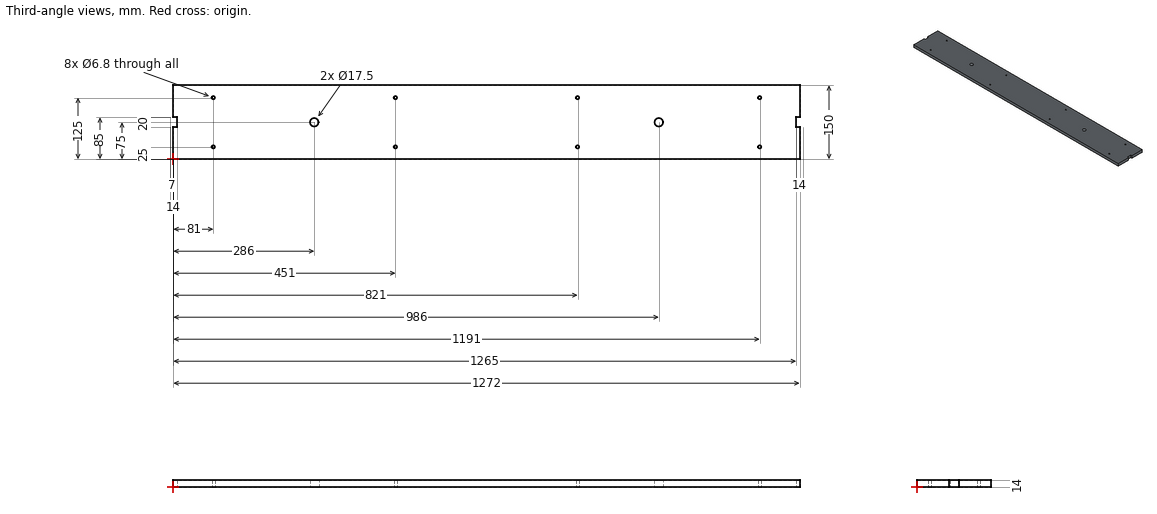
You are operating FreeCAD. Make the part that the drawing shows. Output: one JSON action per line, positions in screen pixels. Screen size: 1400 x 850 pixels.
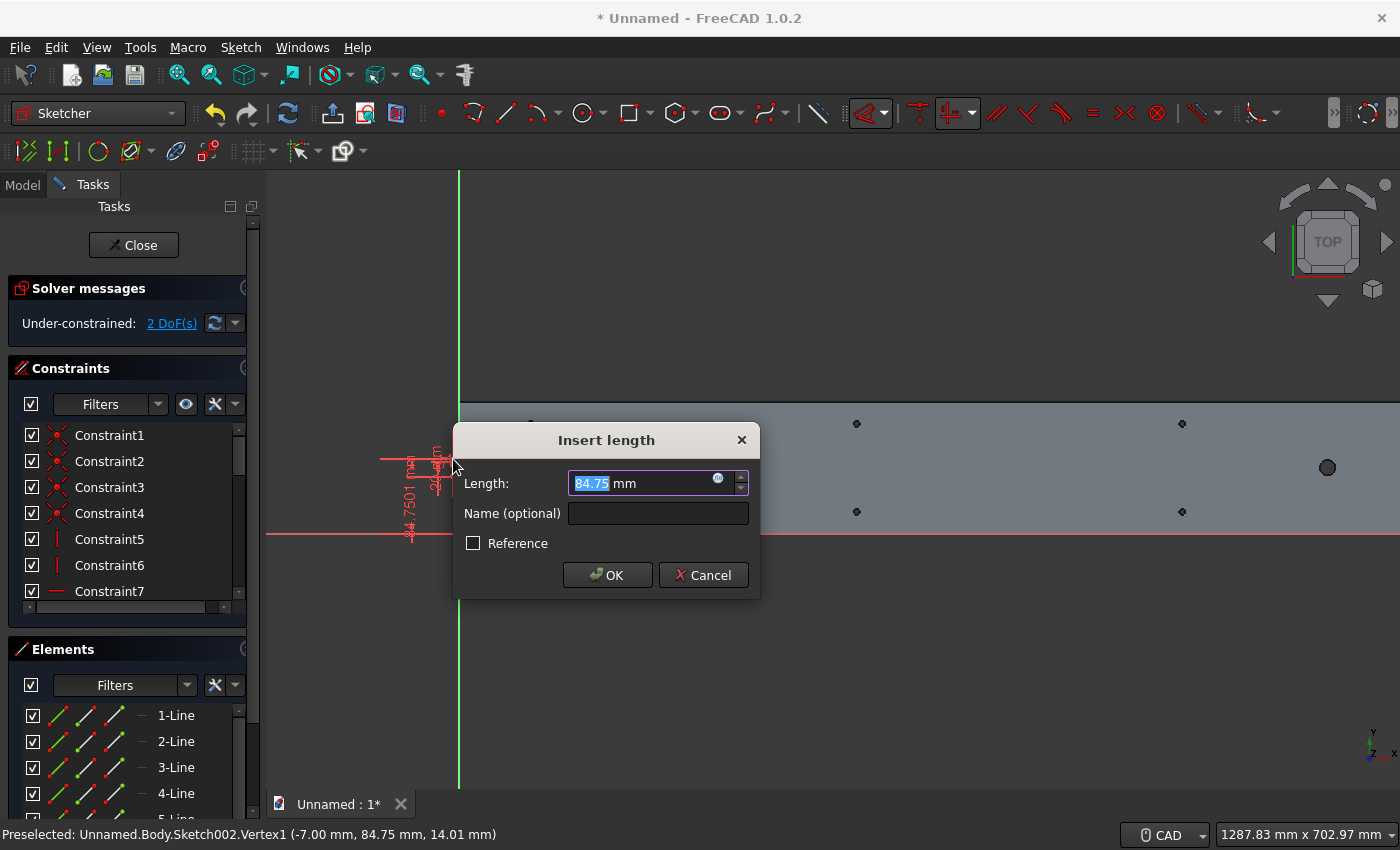
{"action": "type", "text": "85"}
{"action": "key", "text": "Return"}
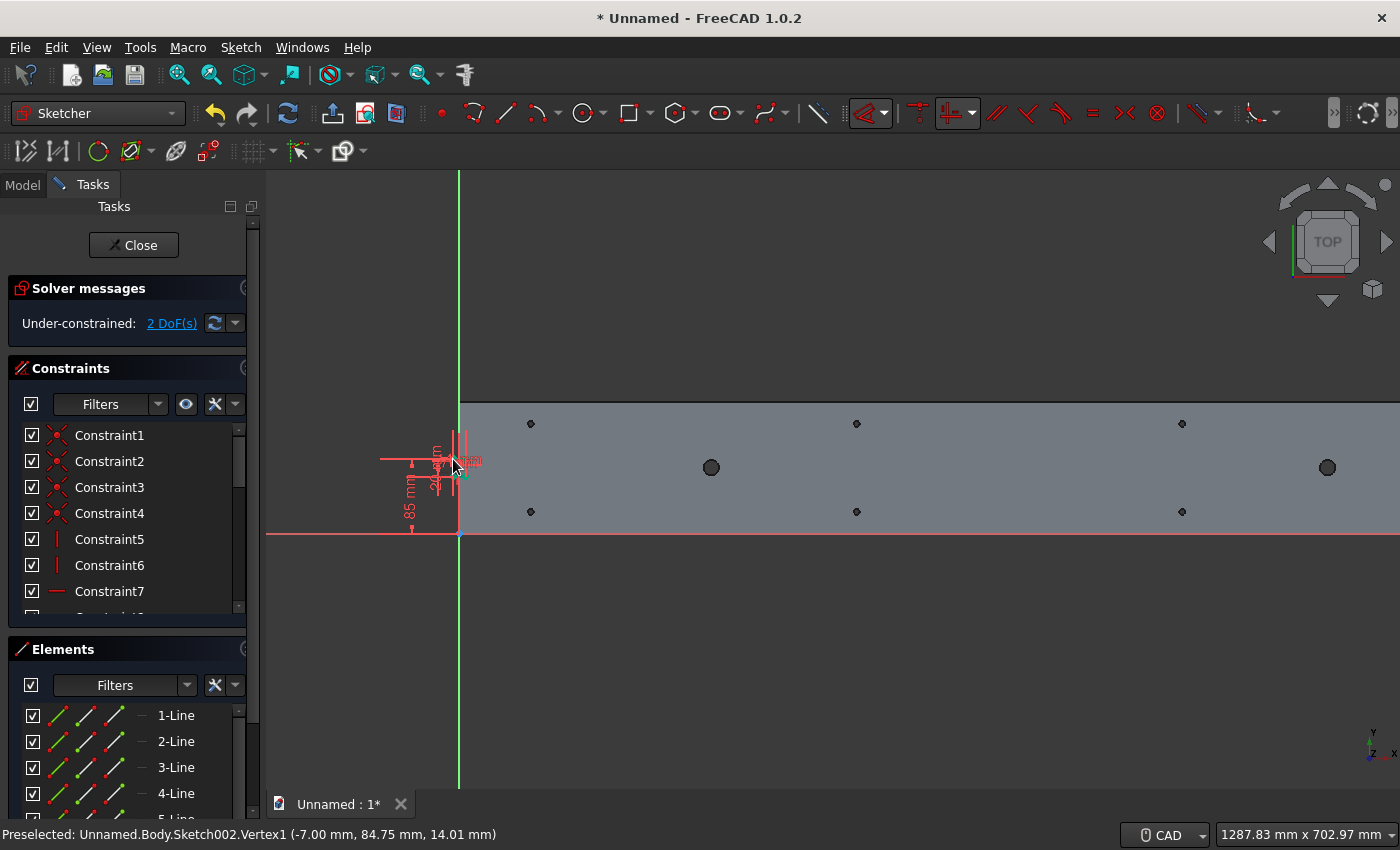
{"action": "scroll", "coordinate": [454, 459], "scroll_direction": "down", "scroll_amount": 3}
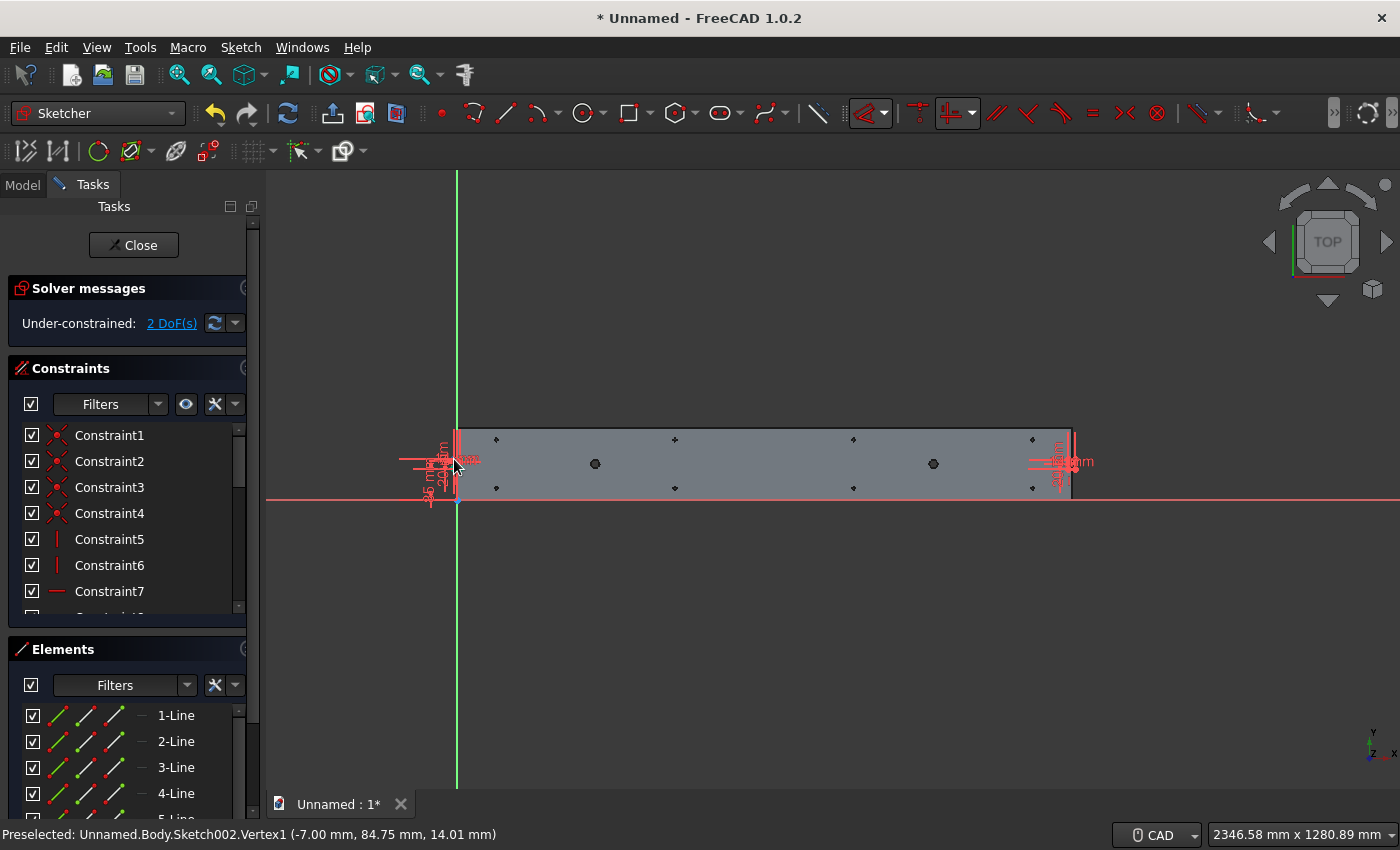
{"action": "scroll", "coordinate": [1068, 460], "scroll_direction": "up", "scroll_amount": 3}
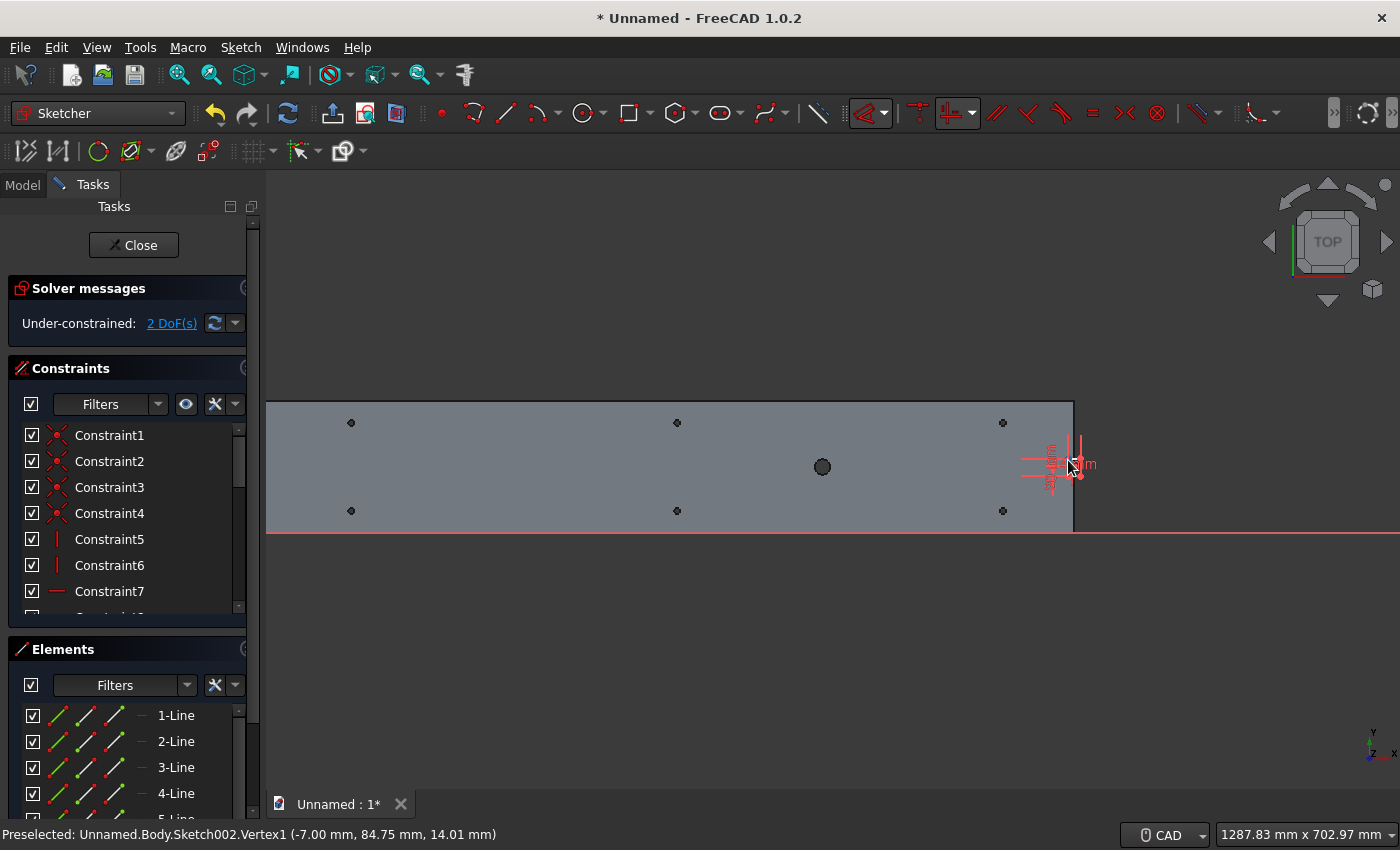
{"action": "left_click", "coordinate": [1068, 459]}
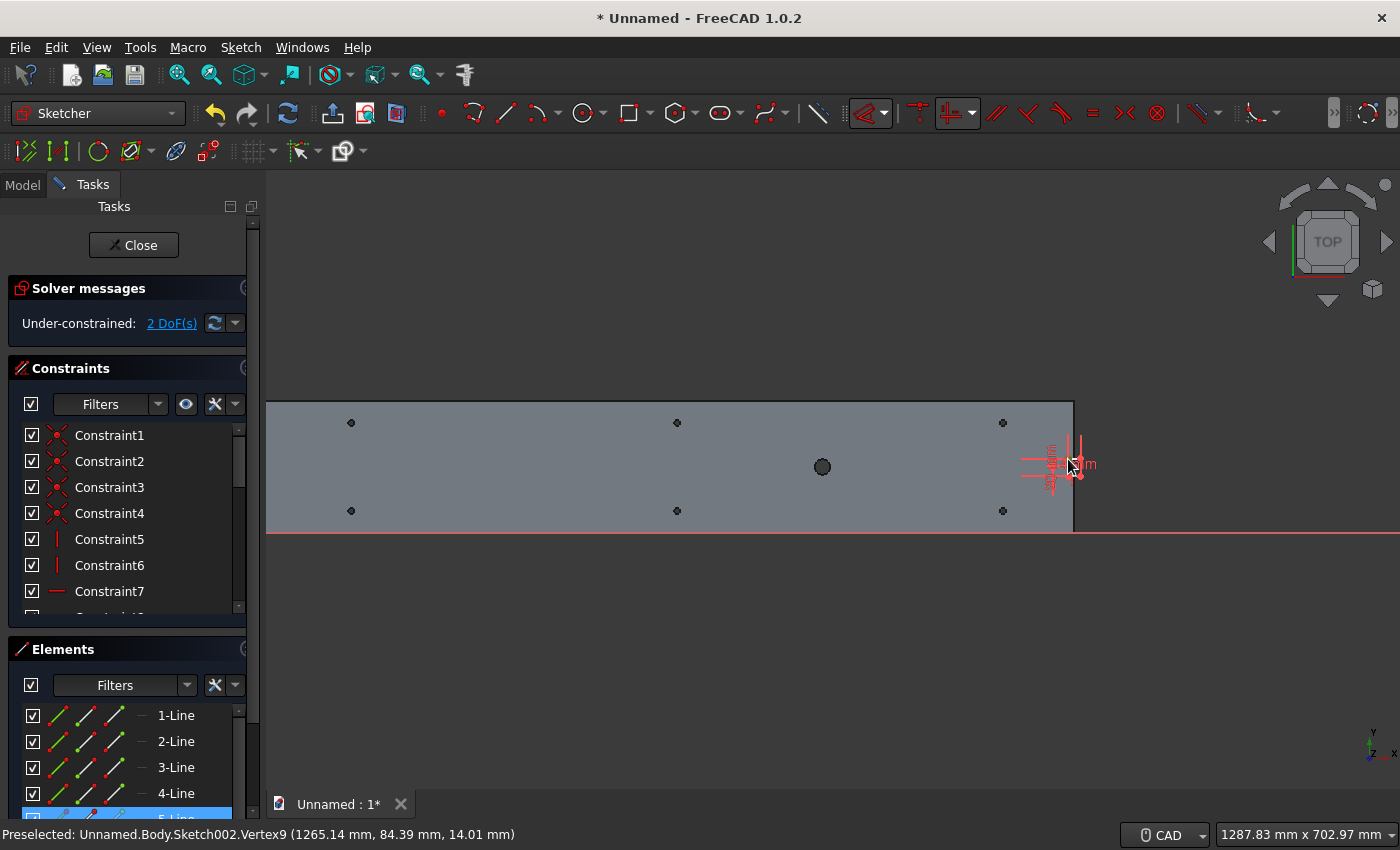
{"action": "left_click", "coordinate": [886, 114]}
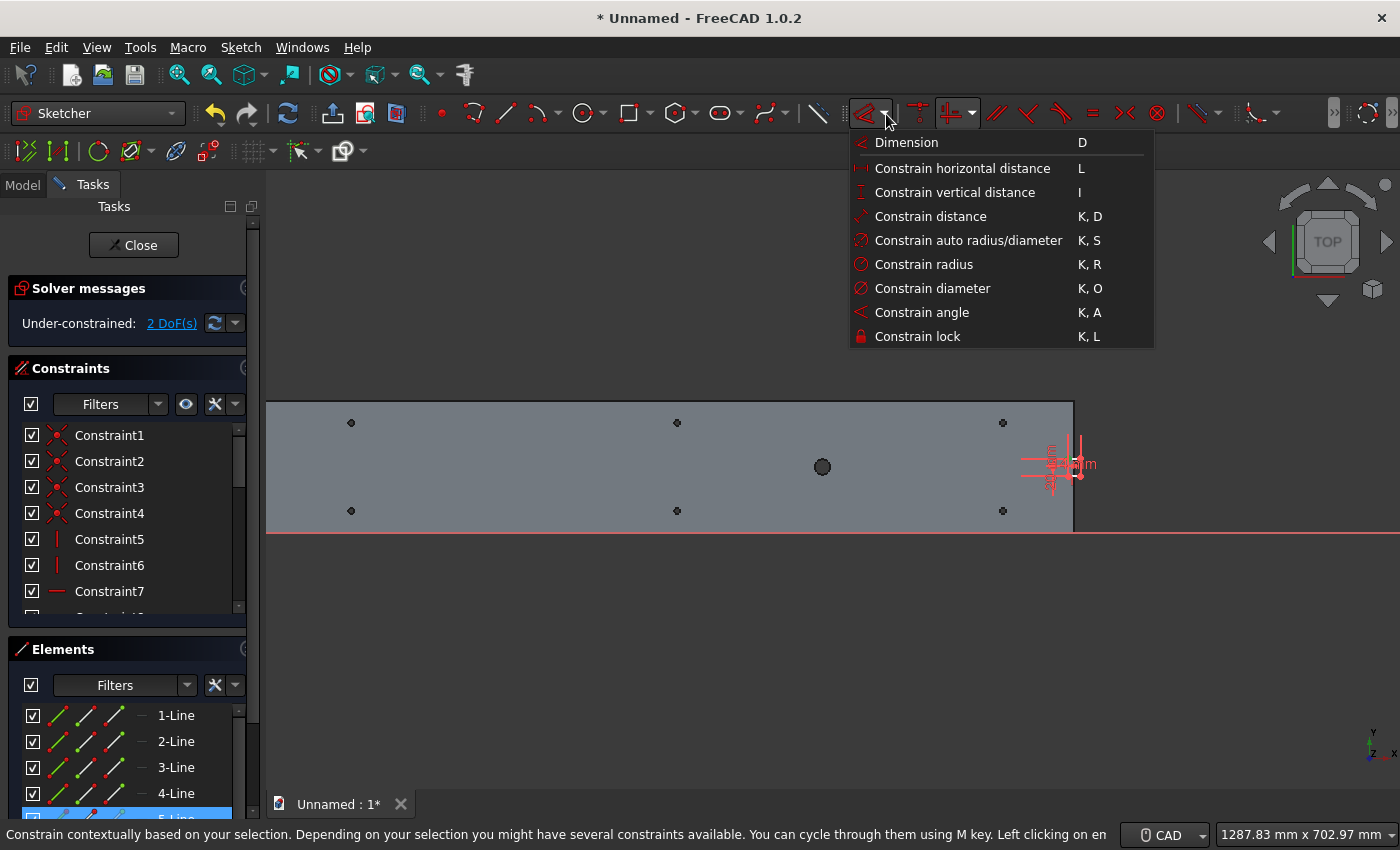
{"action": "left_click", "coordinate": [1002, 192]}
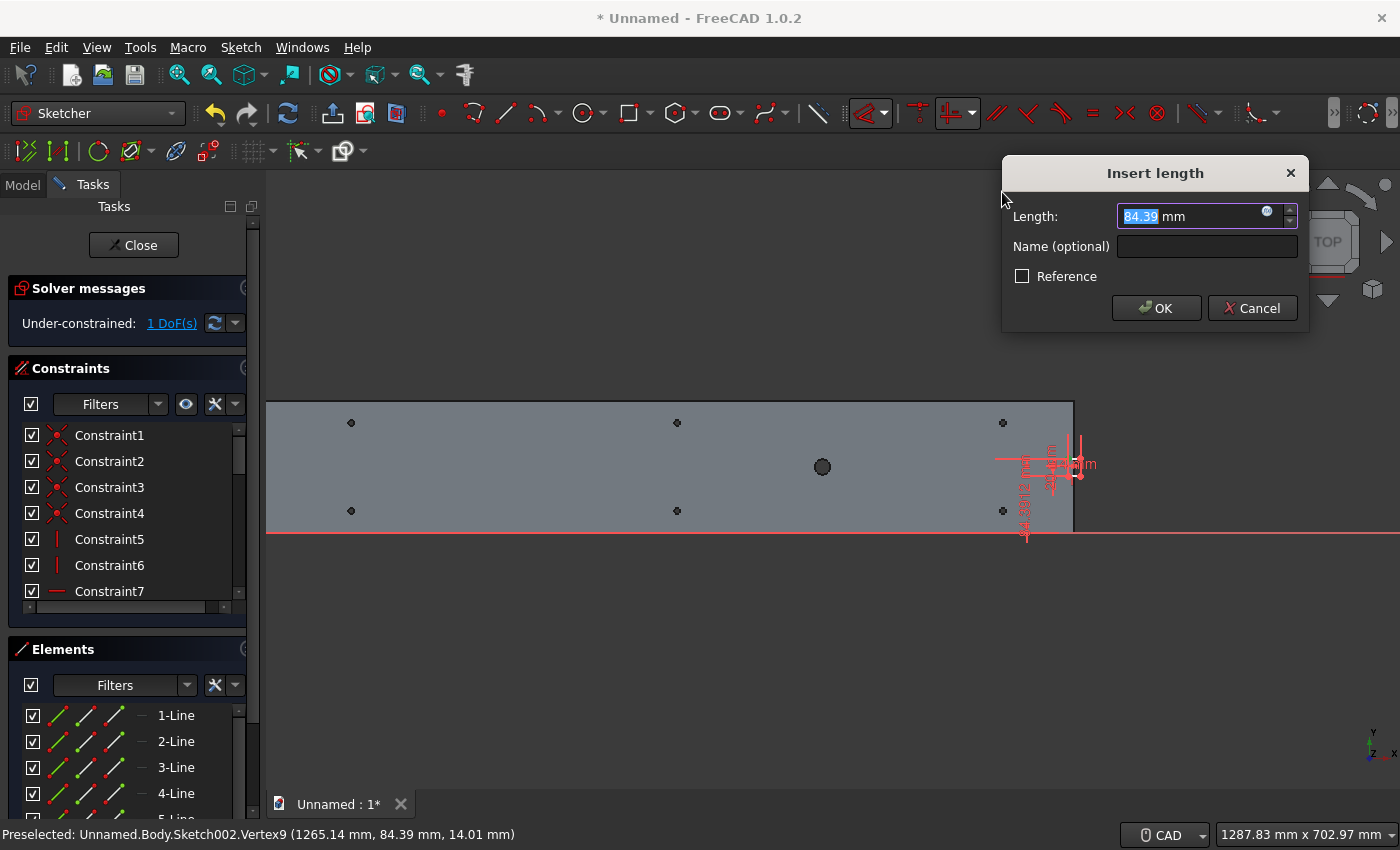
{"action": "type", "text": "85"}
{"action": "key", "text": "Return"}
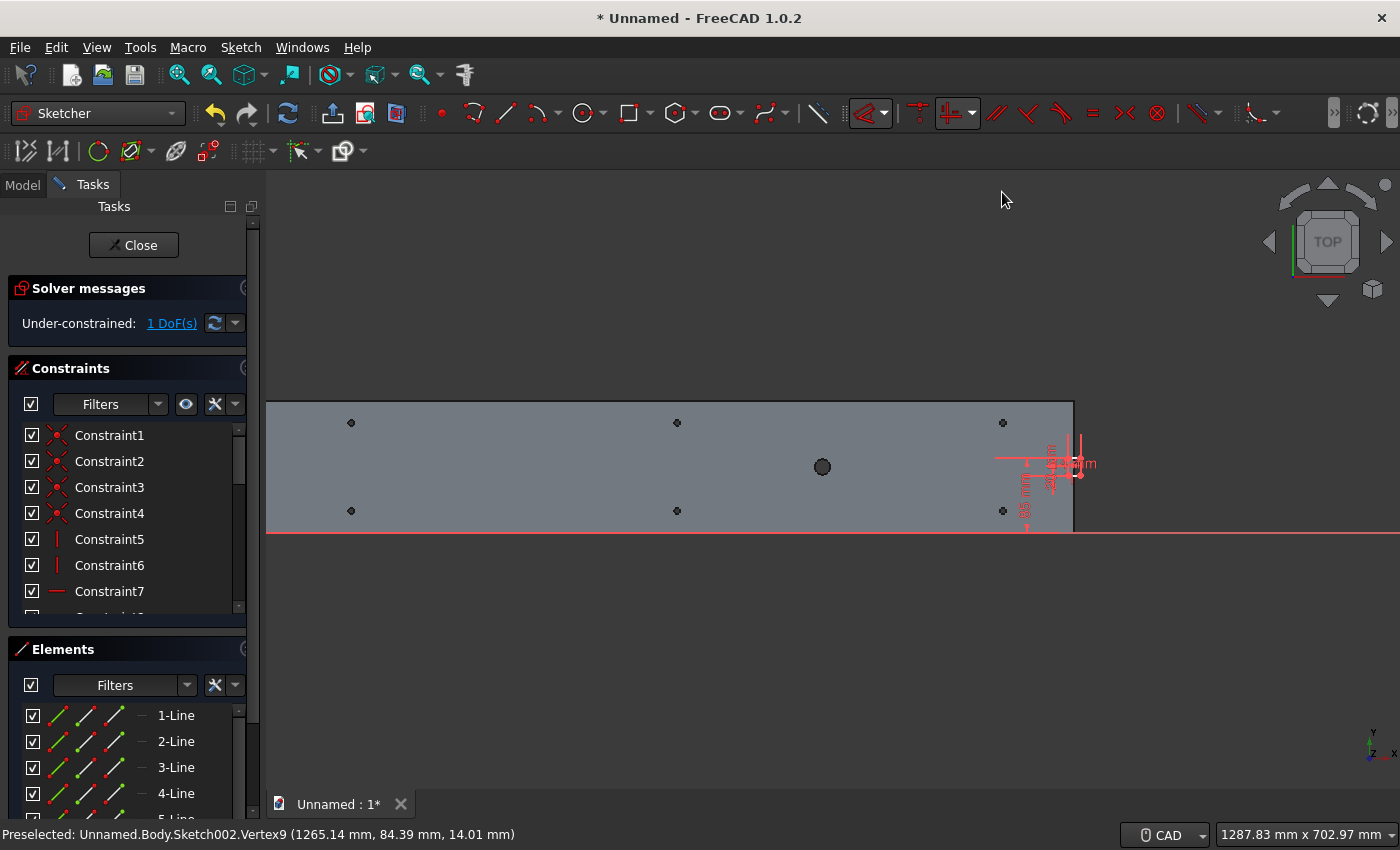
{"action": "left_click", "coordinate": [1068, 458]}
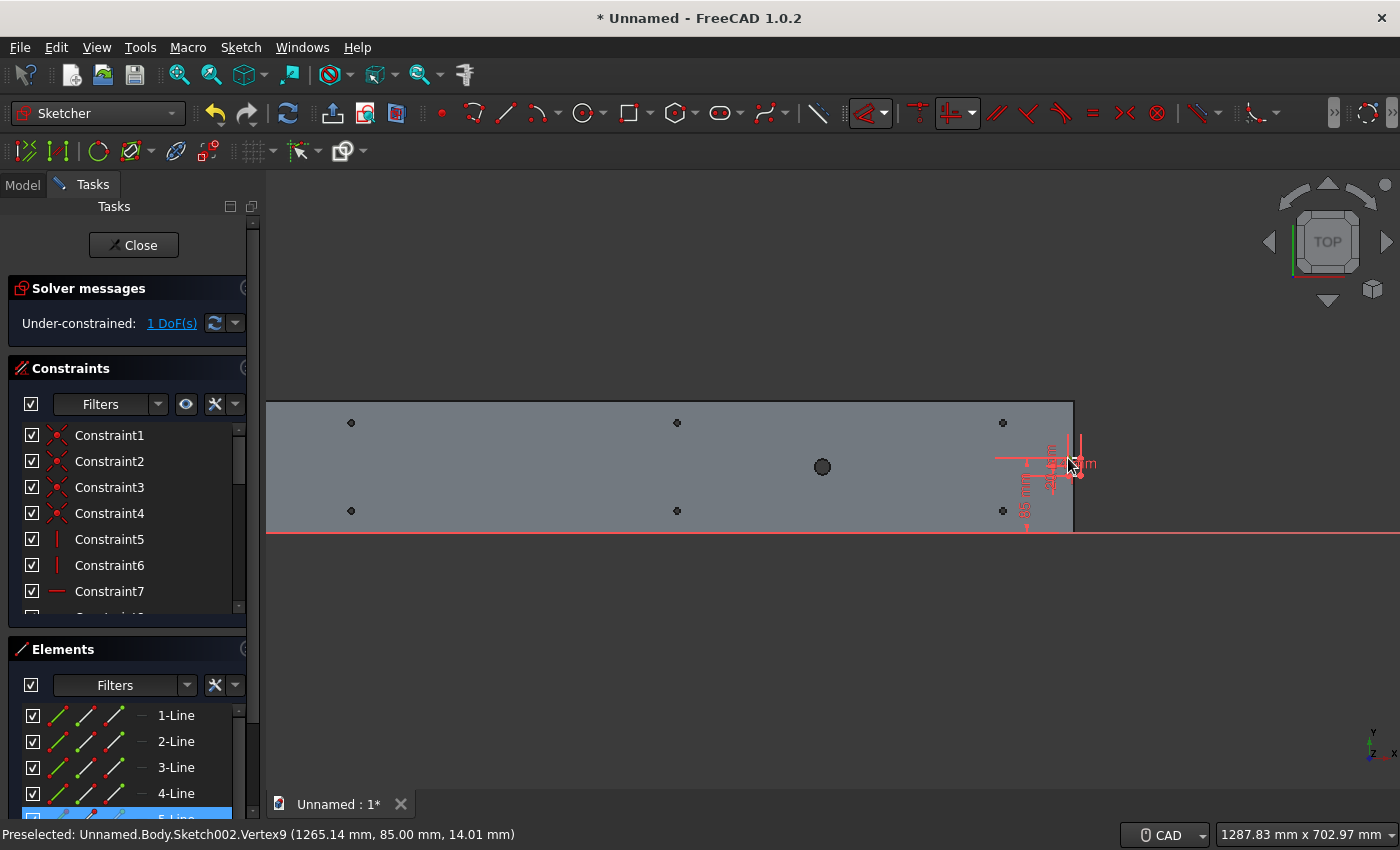
{"action": "left_click", "coordinate": [886, 114]}